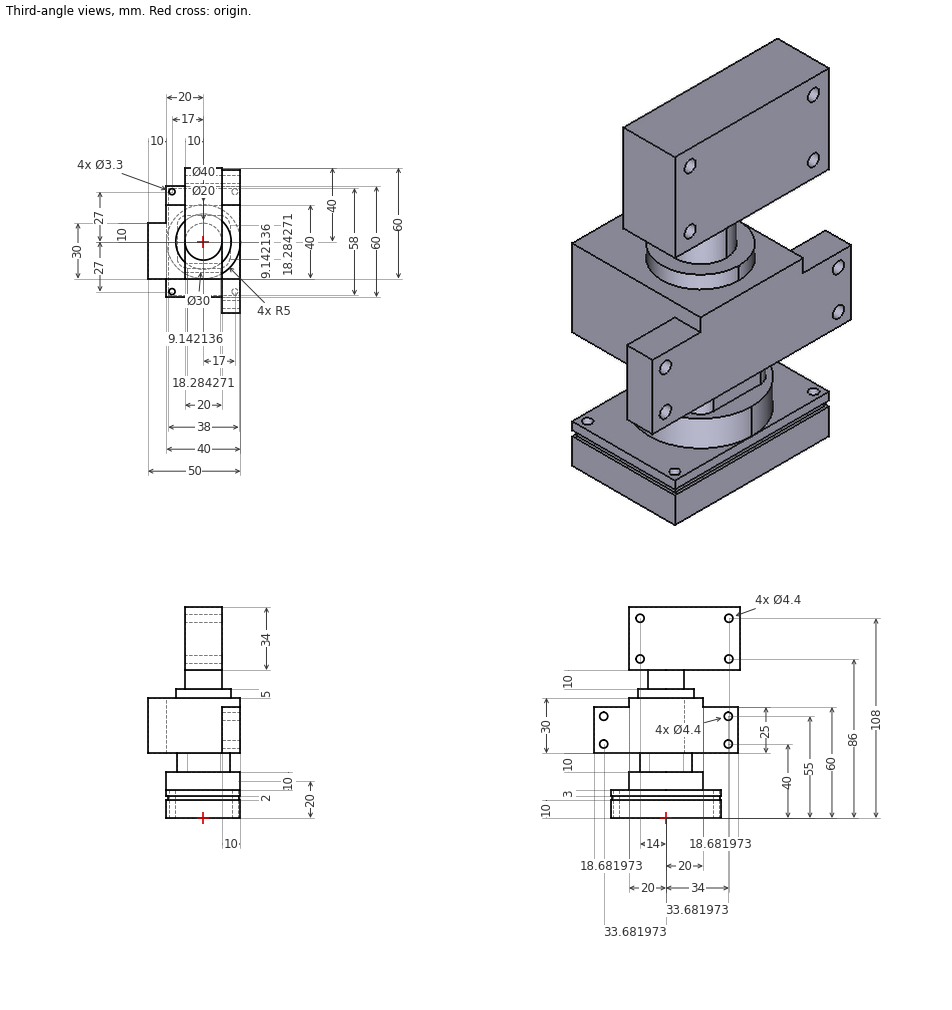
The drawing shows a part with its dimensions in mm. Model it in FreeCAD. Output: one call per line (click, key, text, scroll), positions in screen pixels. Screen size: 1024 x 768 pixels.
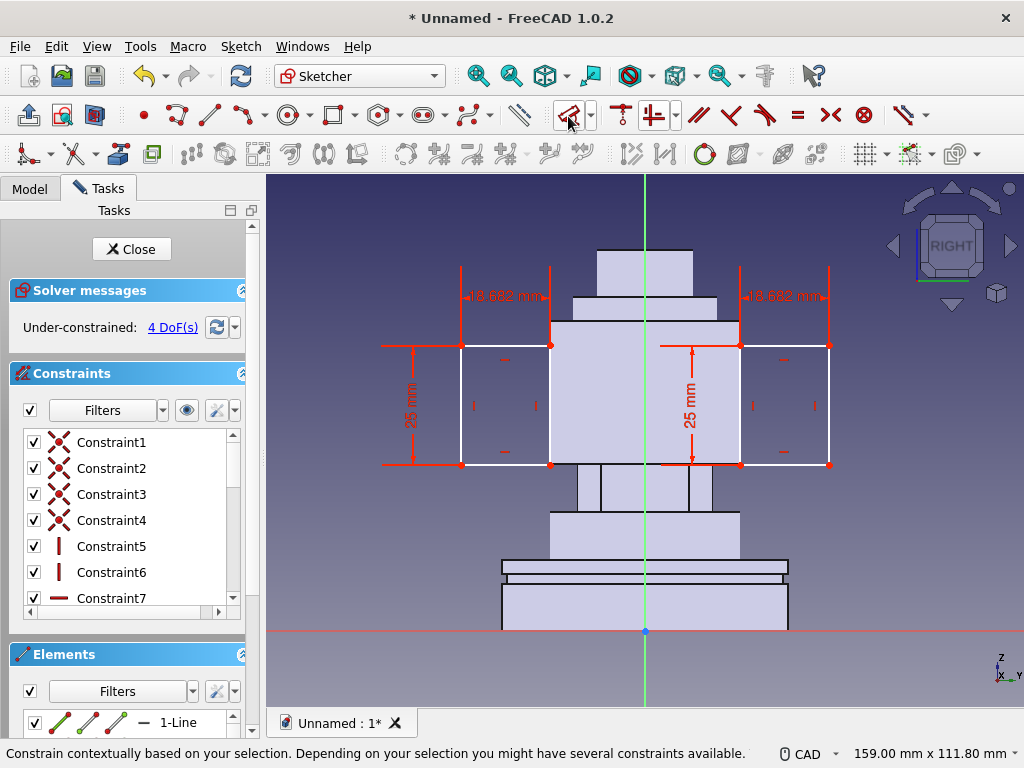
click(740, 346)
click(692, 665)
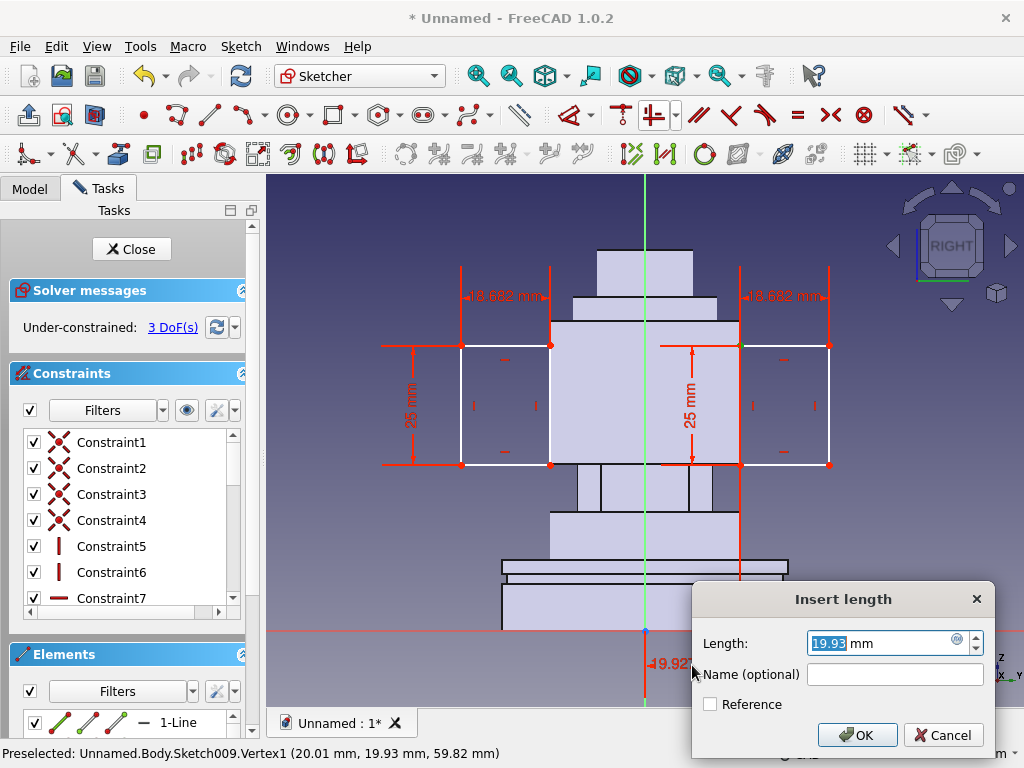
text(20)
key(Return)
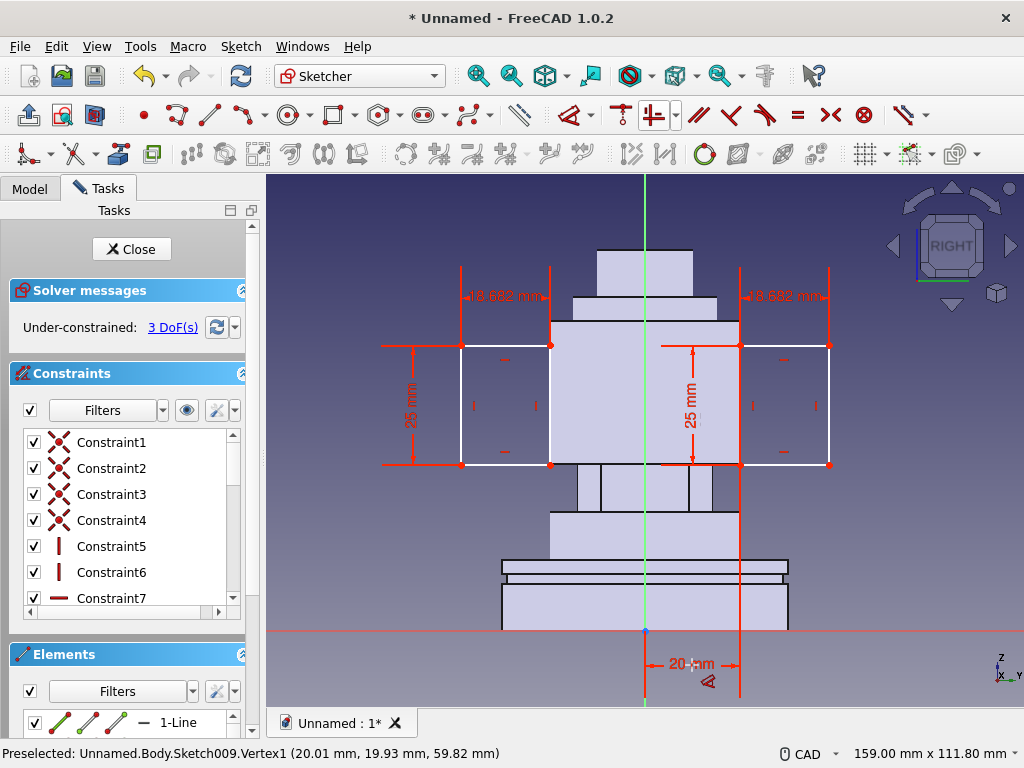
click(740, 346)
click(774, 489)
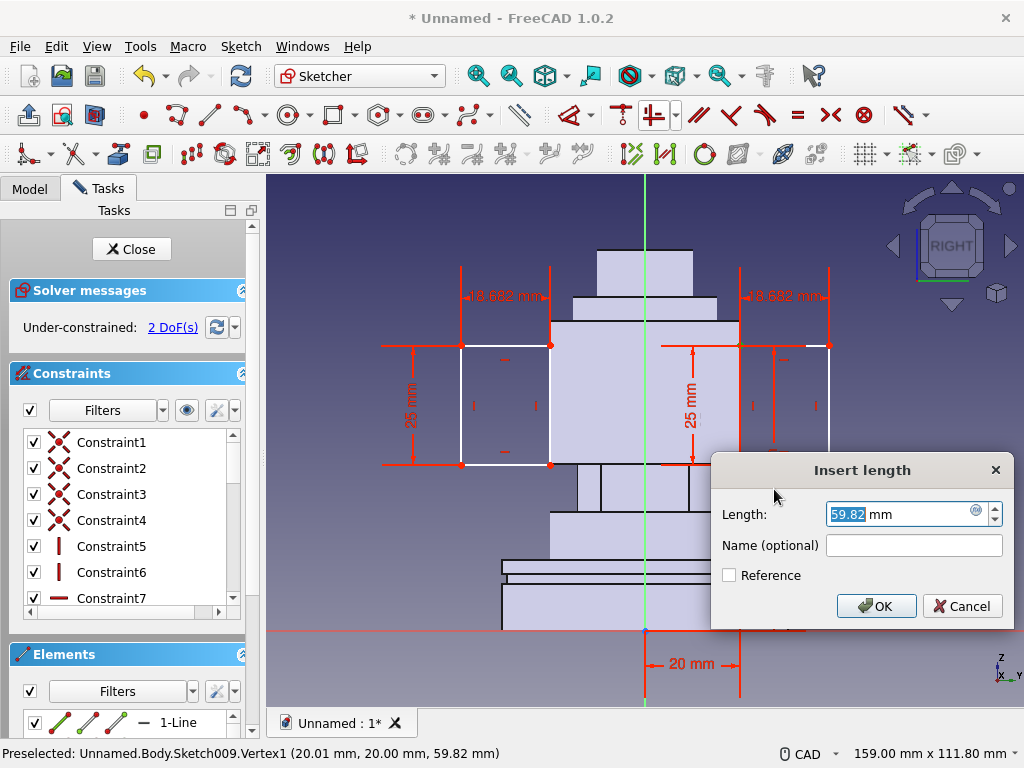
text(60)
key(Return)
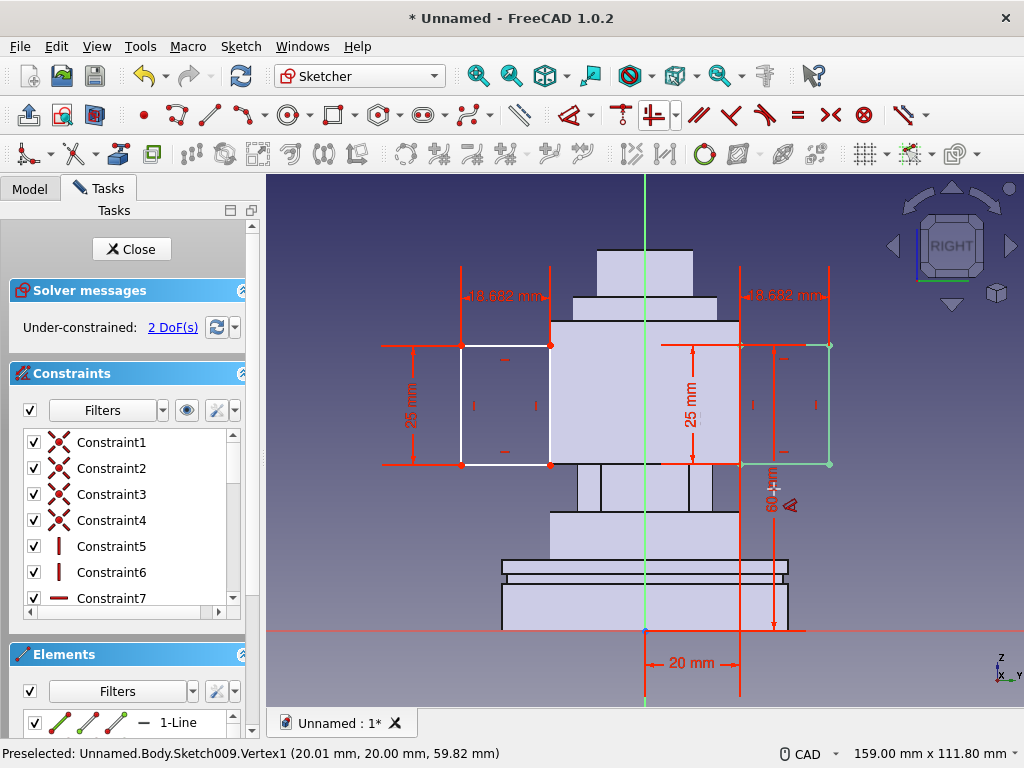
click(461, 346)
click(427, 489)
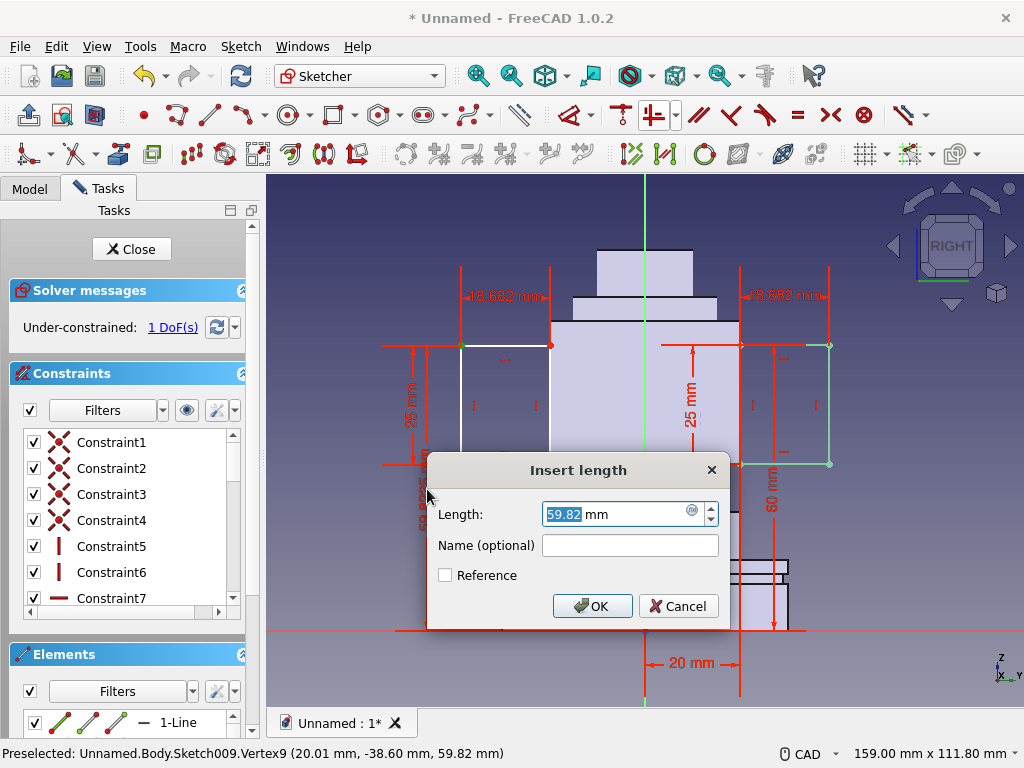
text(60)
key(Return)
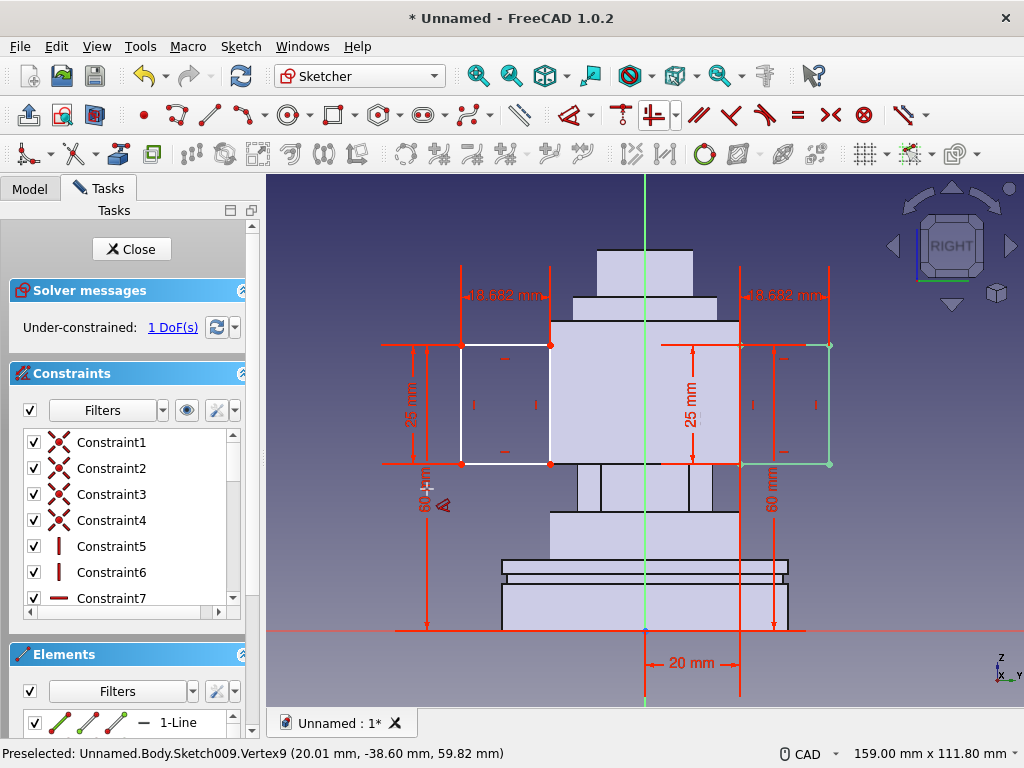
click(550, 464)
click(598, 665)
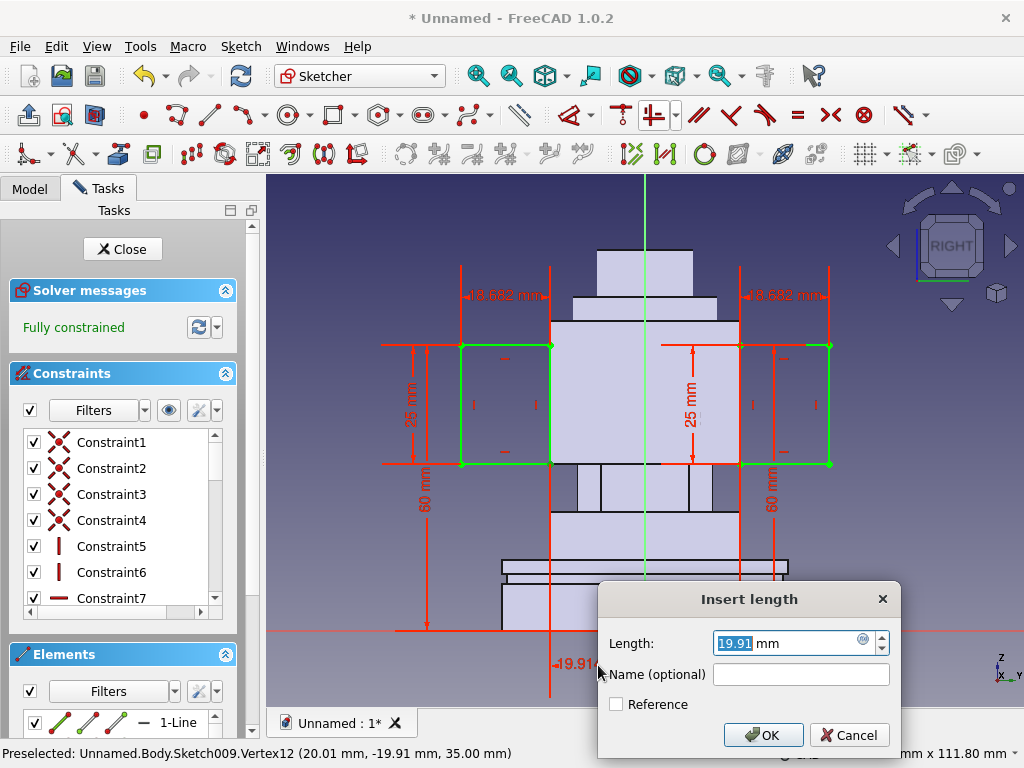
text(20)
key(Return)
key(Escape)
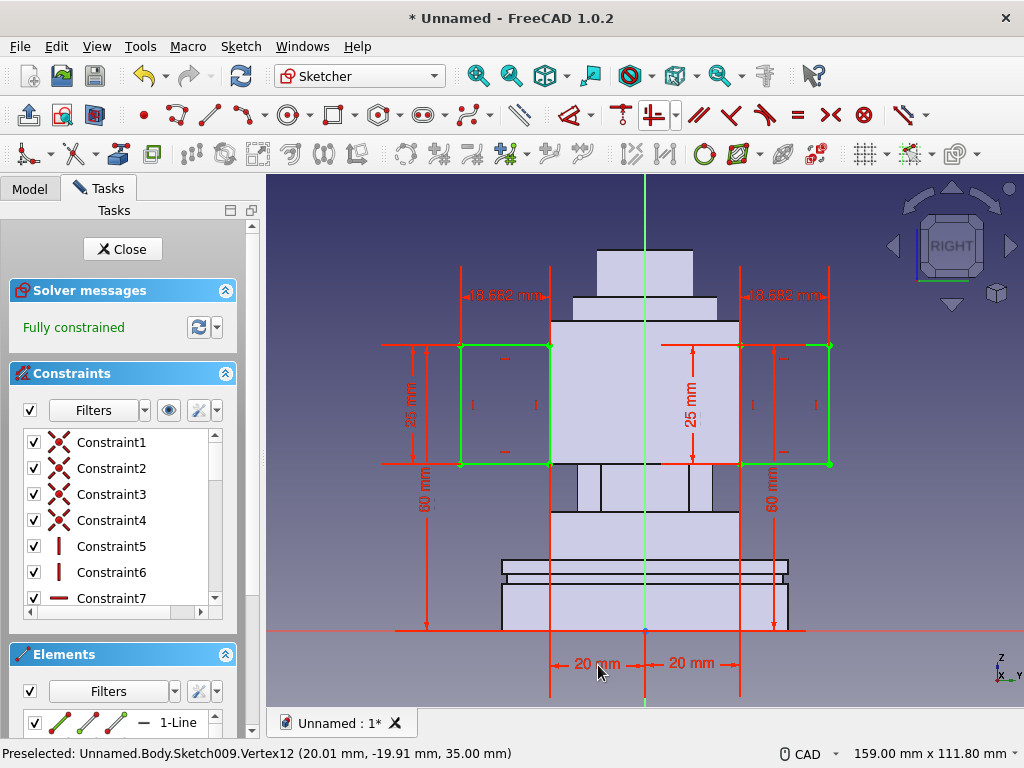
click(123, 249)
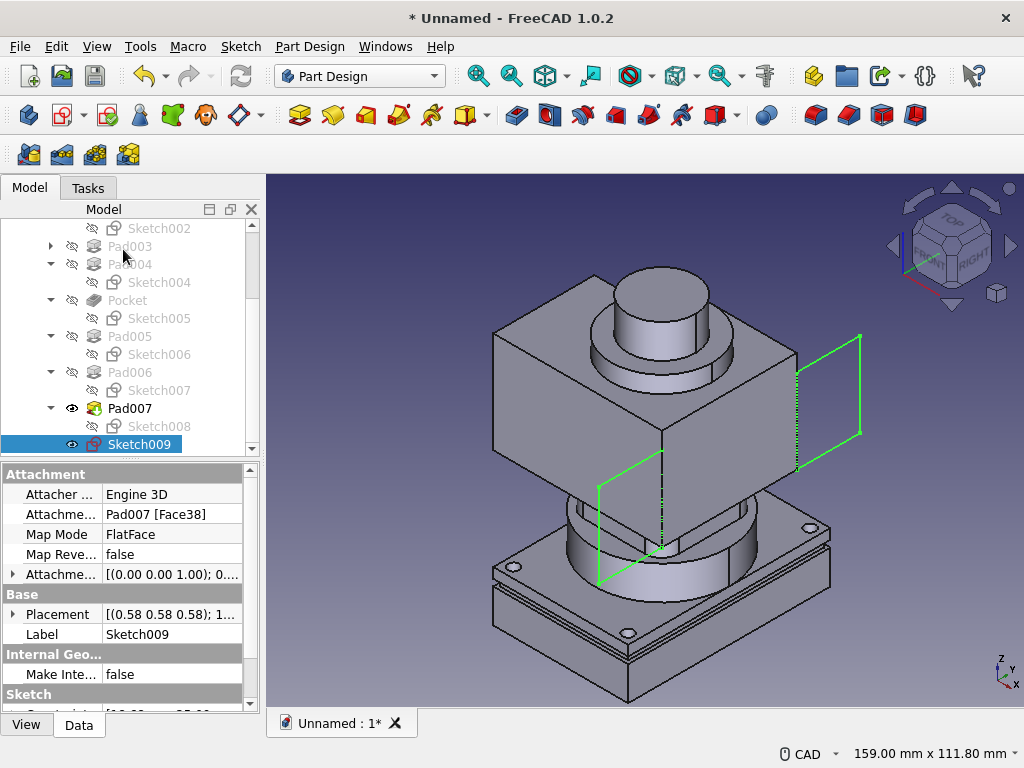
click(300, 116)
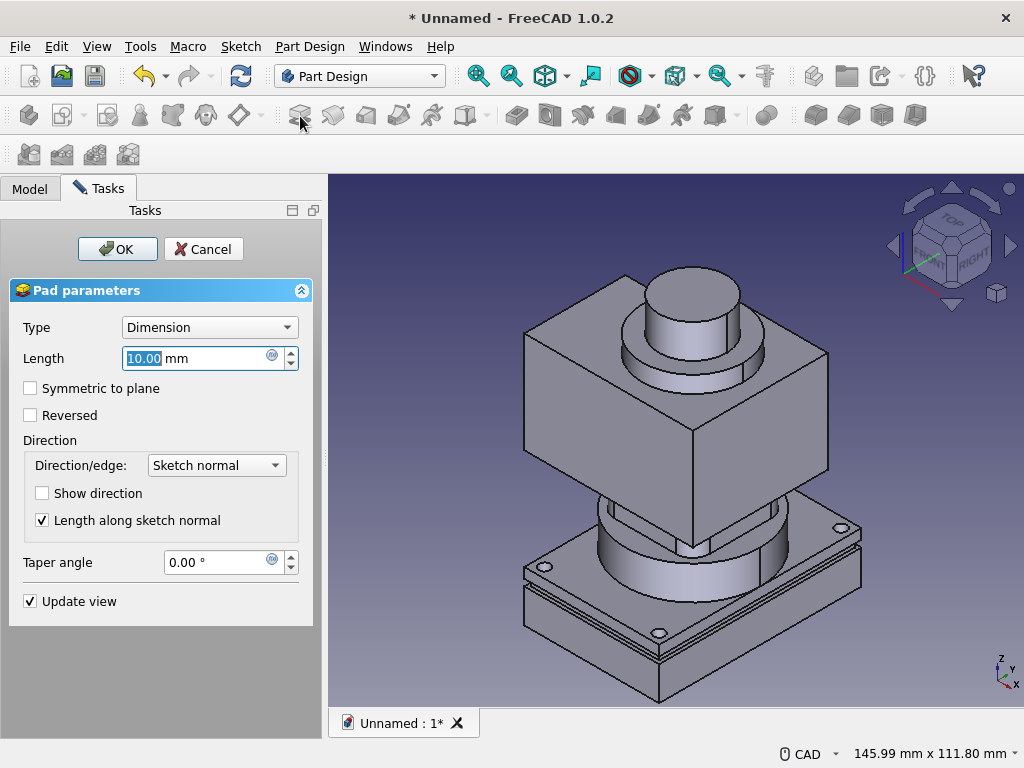
text(10)
key(Tab)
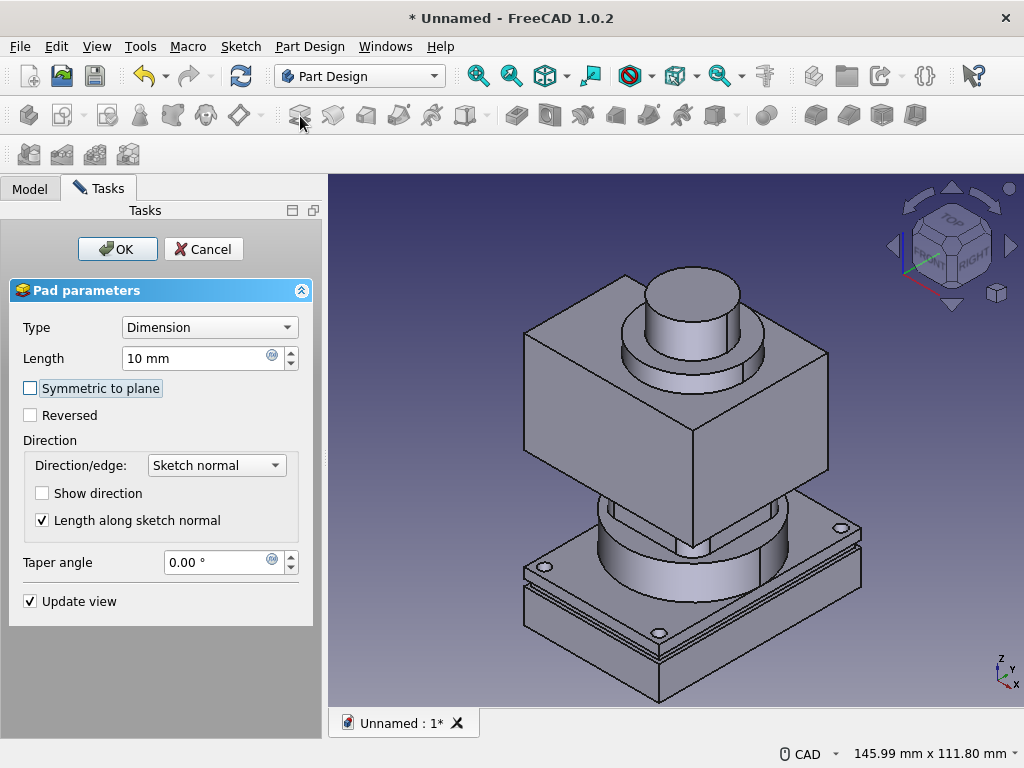
click(31, 415)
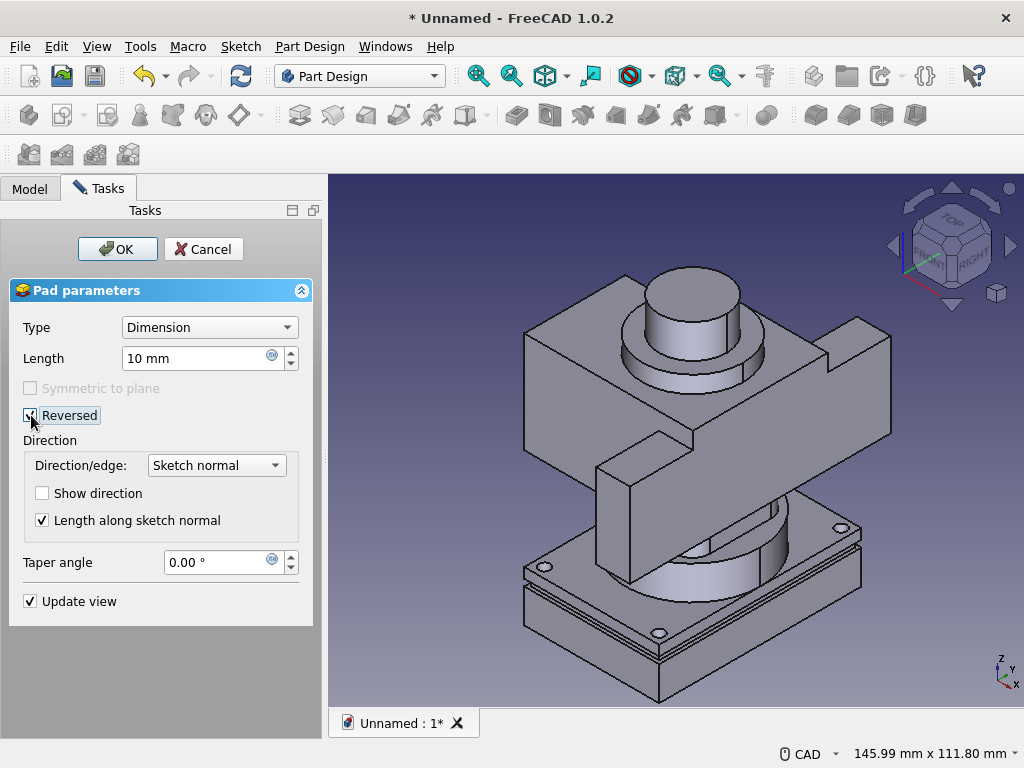
click(118, 249)